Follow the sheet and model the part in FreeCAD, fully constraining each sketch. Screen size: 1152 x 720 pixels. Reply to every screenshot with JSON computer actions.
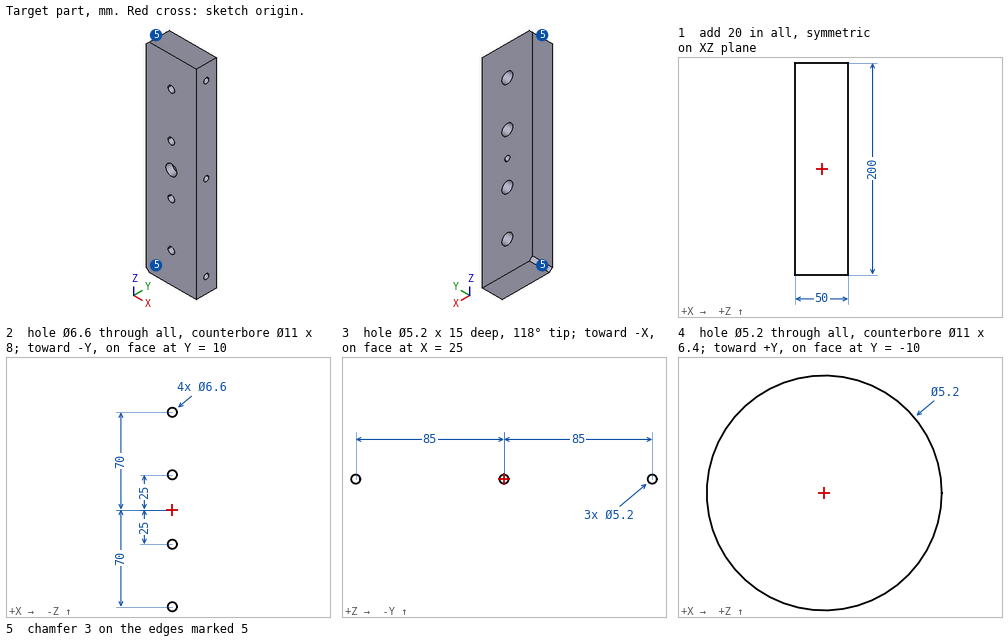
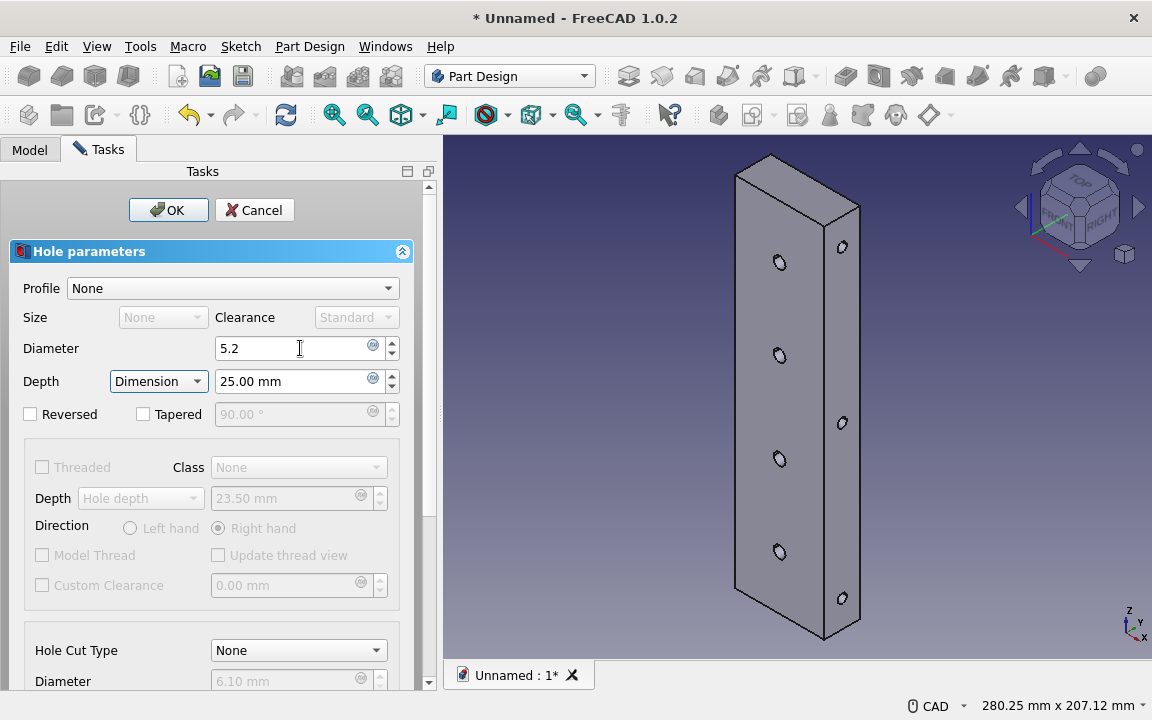
{"action": "triple_click", "coordinate": [300, 382]}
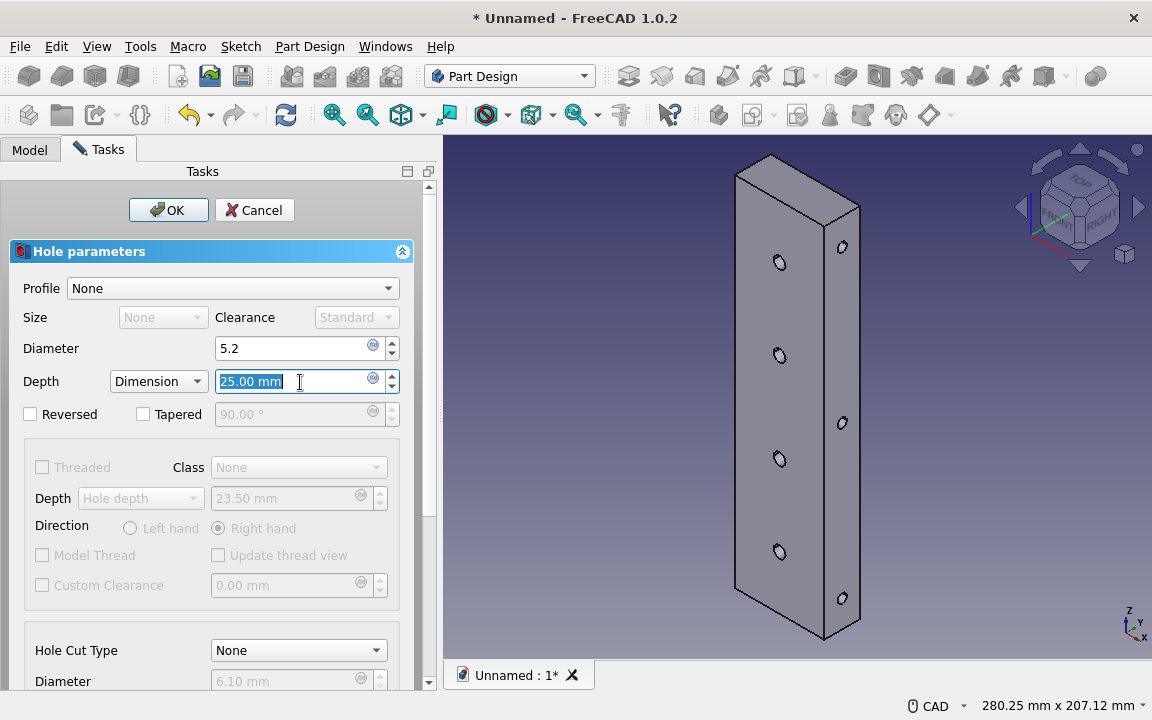
{"action": "type", "text": "15"}
{"action": "key", "text": "Tab"}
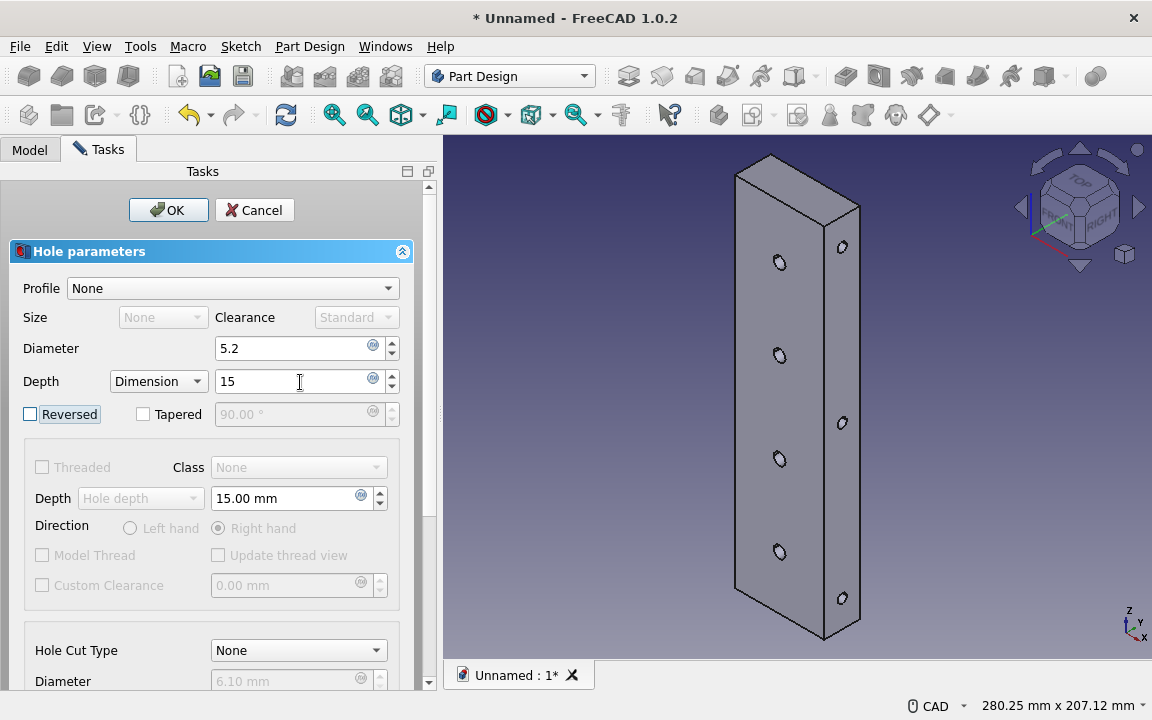
{"action": "left_click", "coordinate": [169, 210]}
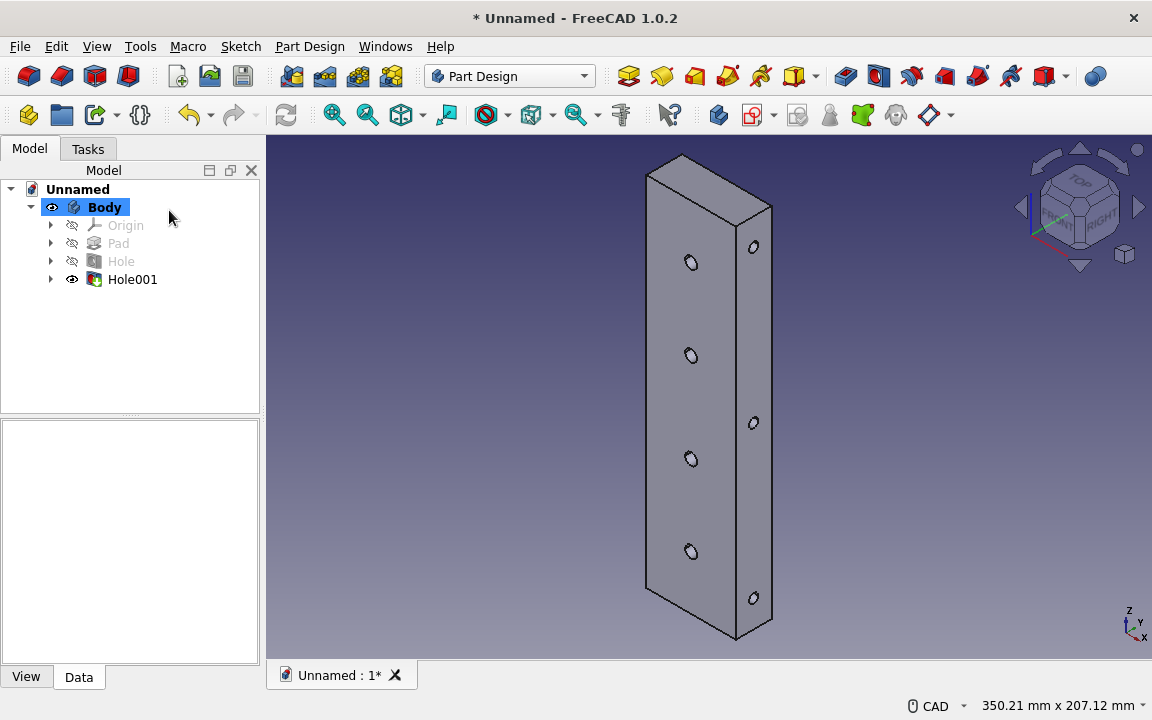
{"action": "left_click", "coordinate": [691, 406]}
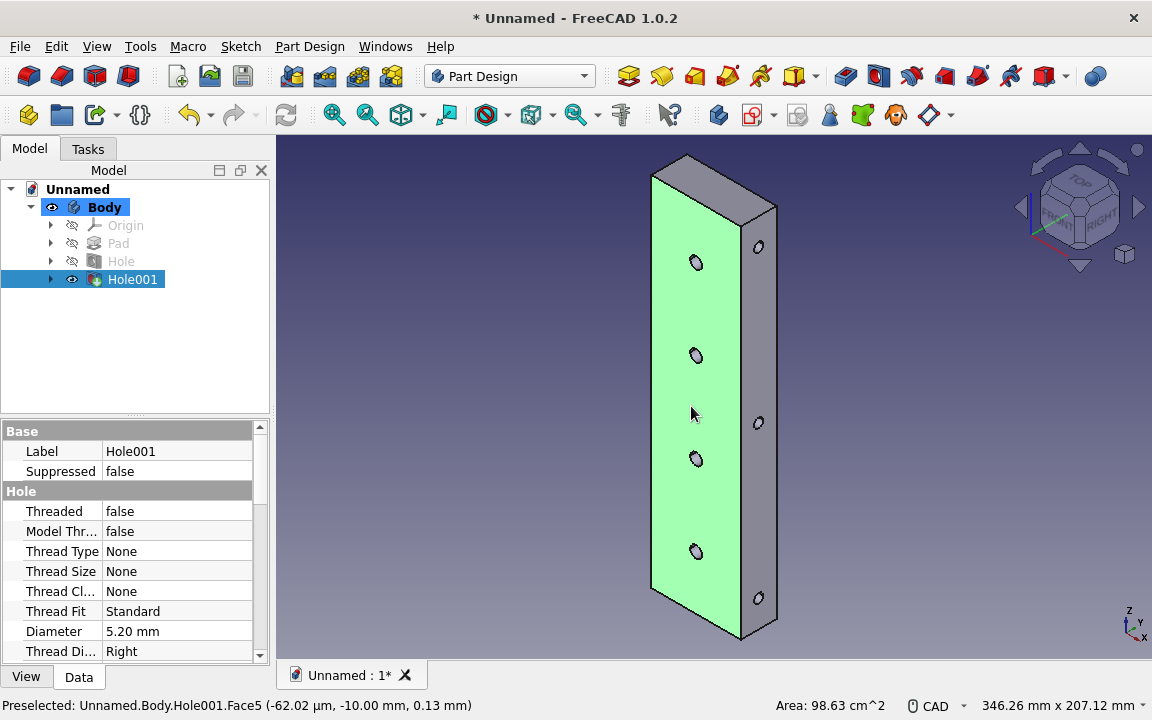
{"action": "left_click", "coordinate": [752, 116]}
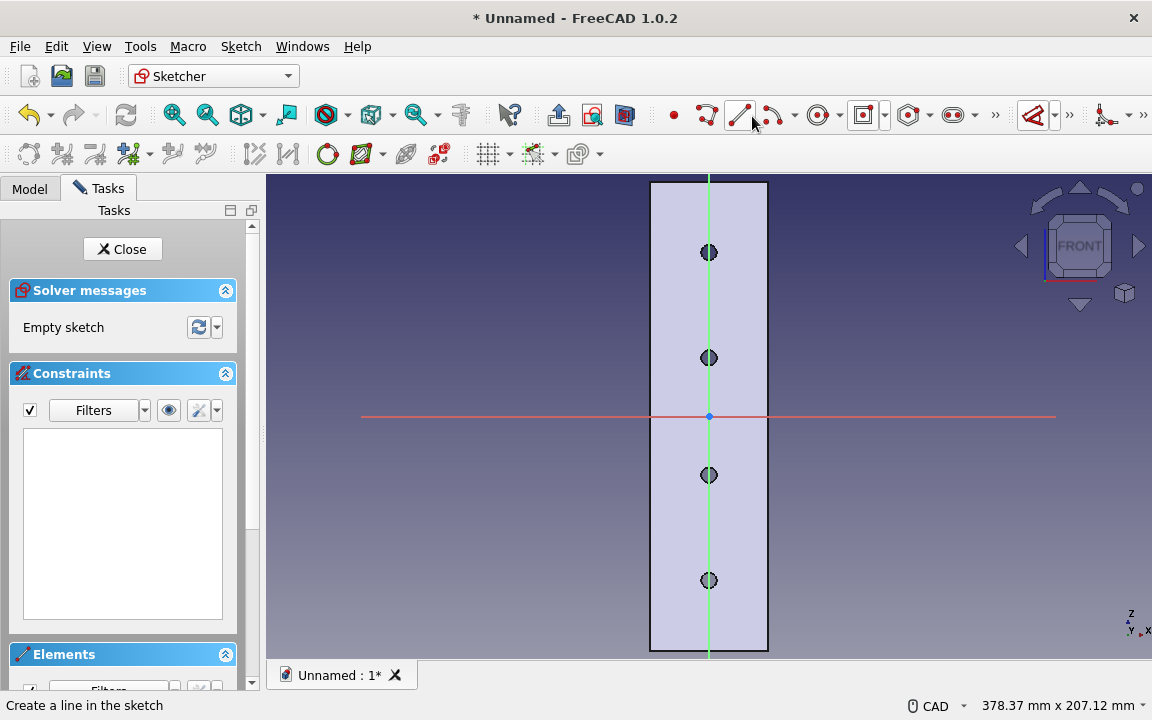
{"action": "scroll", "coordinate": [713, 417], "scroll_direction": "up", "scroll_amount": 15}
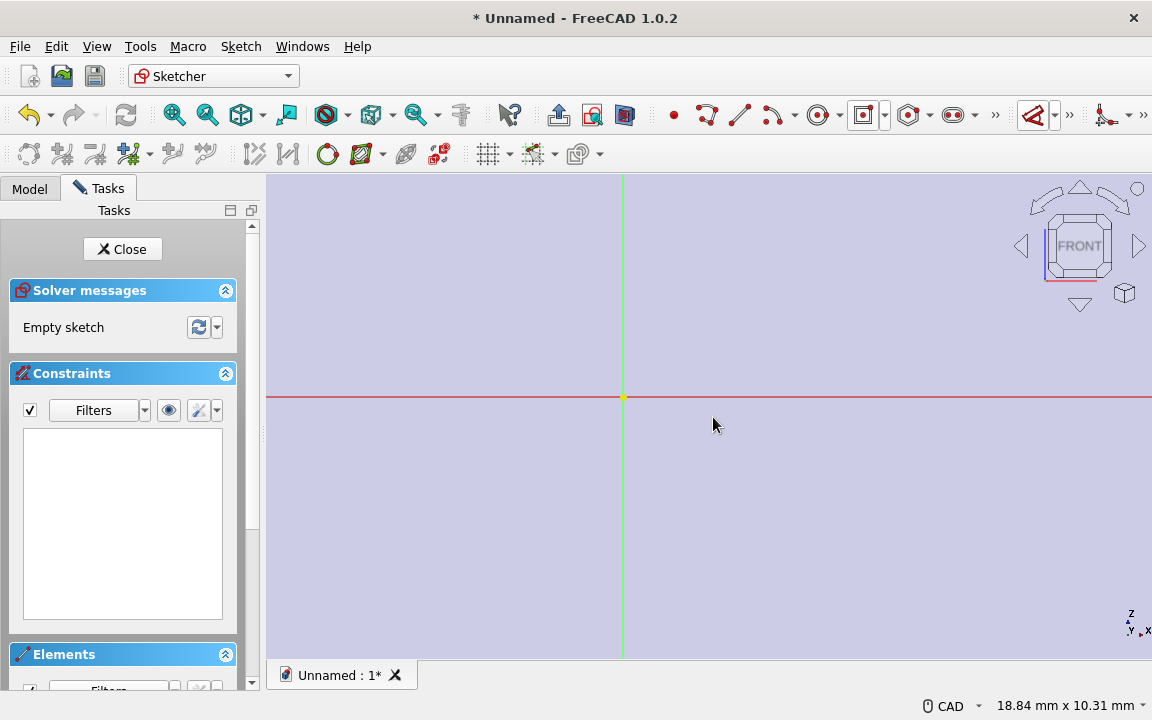
{"action": "left_click", "coordinate": [818, 116]}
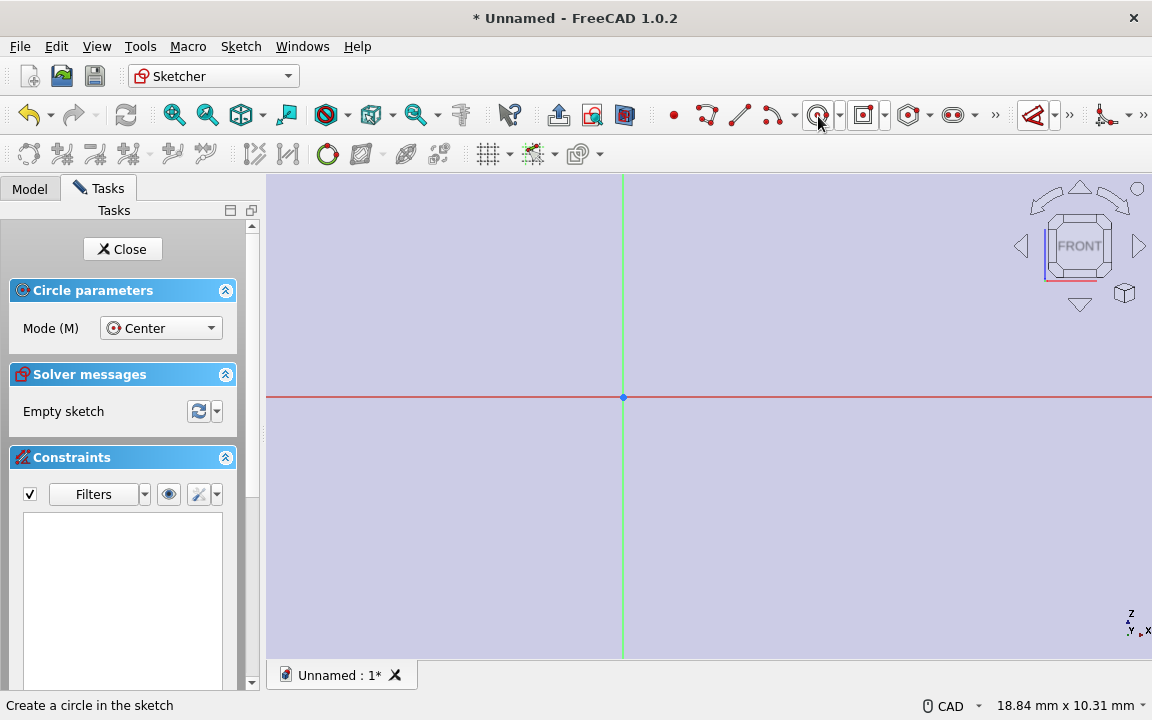
{"action": "left_click", "coordinate": [623, 397]}
{"action": "left_click", "coordinate": [709, 311]}
{"action": "key", "text": "Escape"}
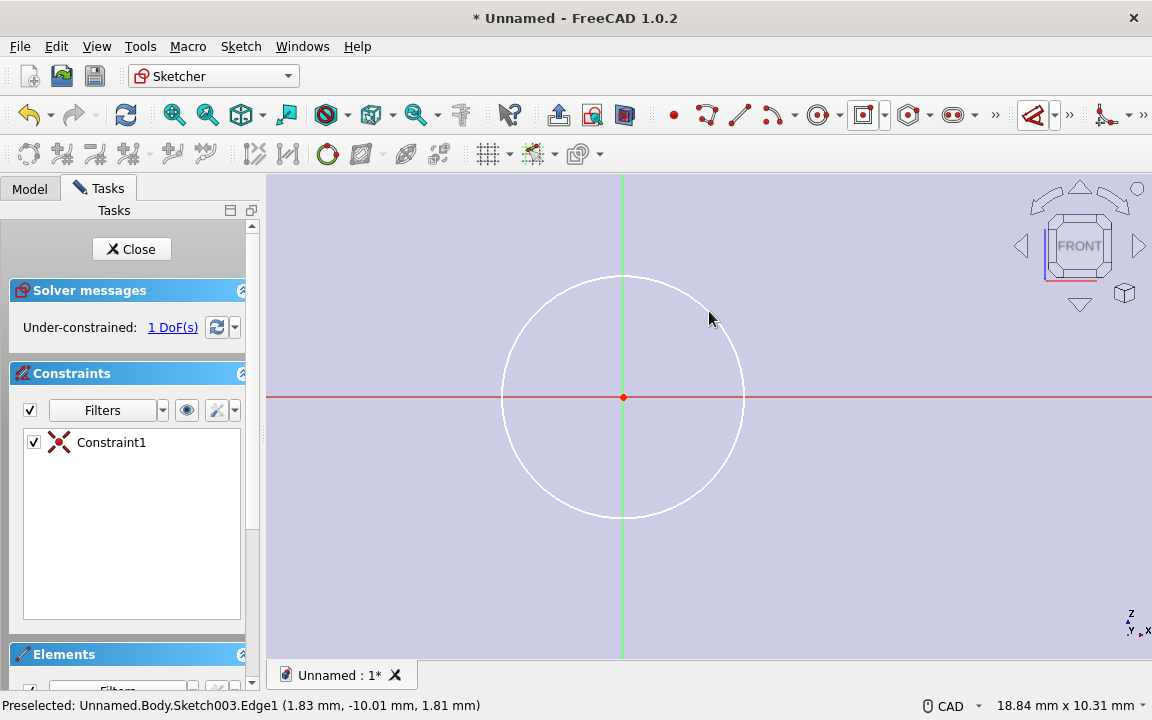
{"action": "left_click", "coordinate": [708, 311]}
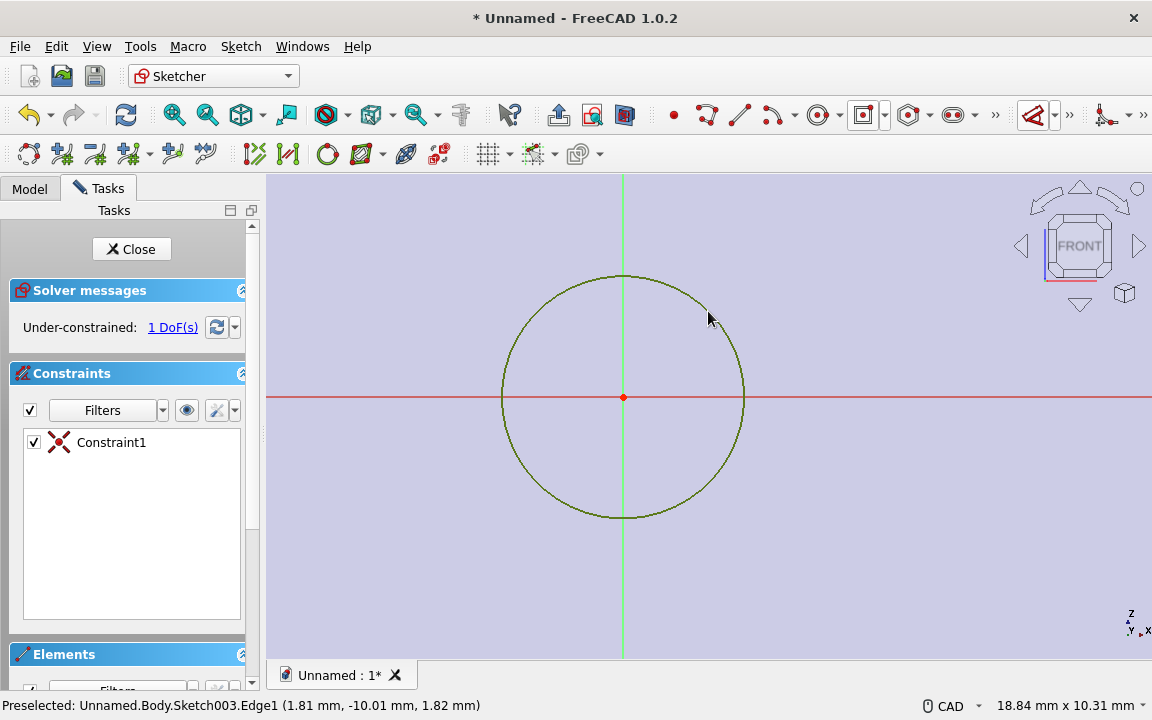
{"action": "key", "text": "k o"}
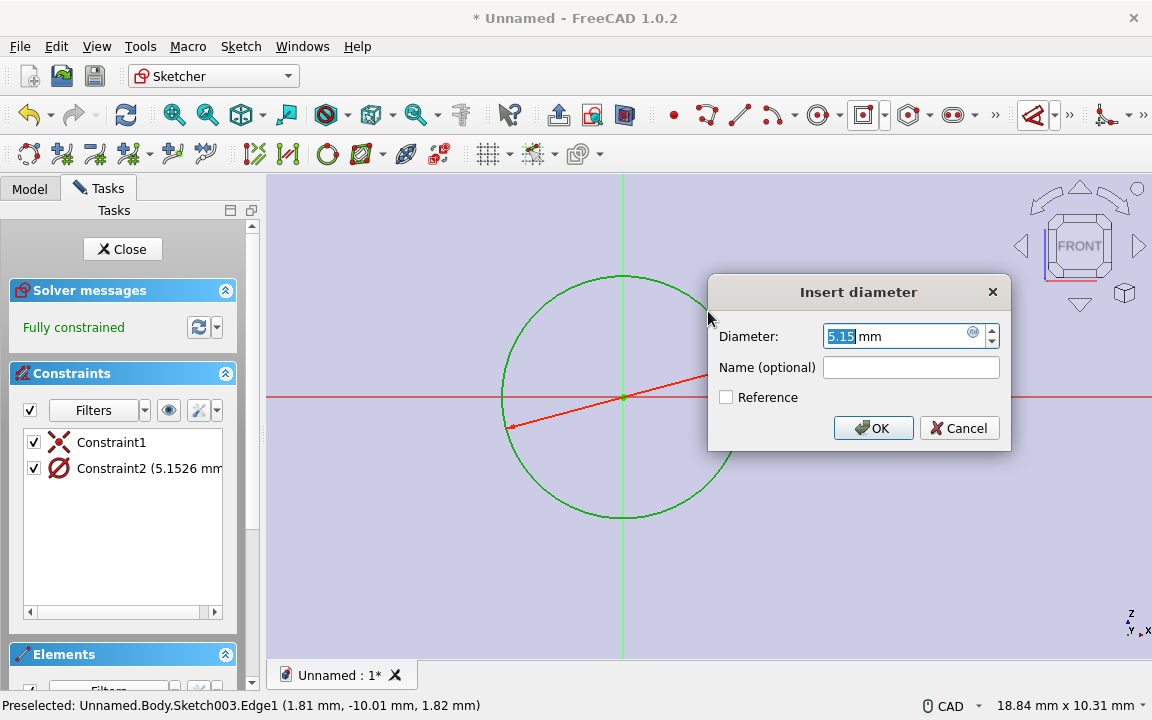
{"action": "type", "text": "5.2"}
{"action": "key", "text": "Return"}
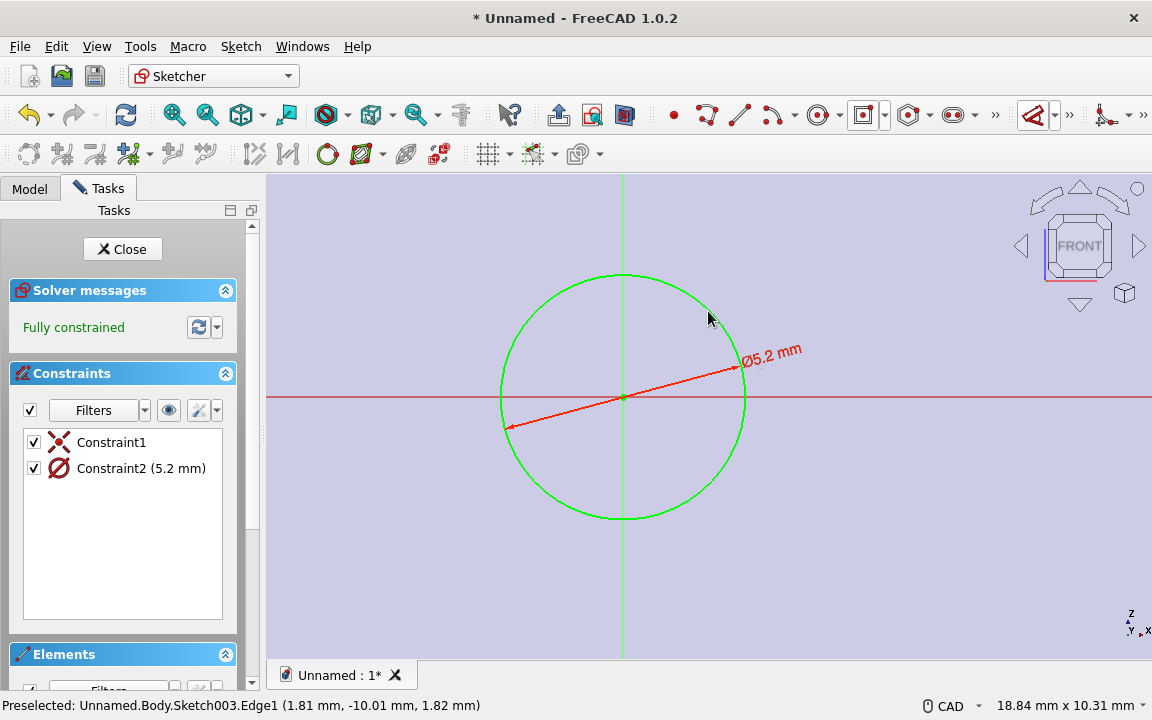
{"action": "left_click", "coordinate": [123, 249]}